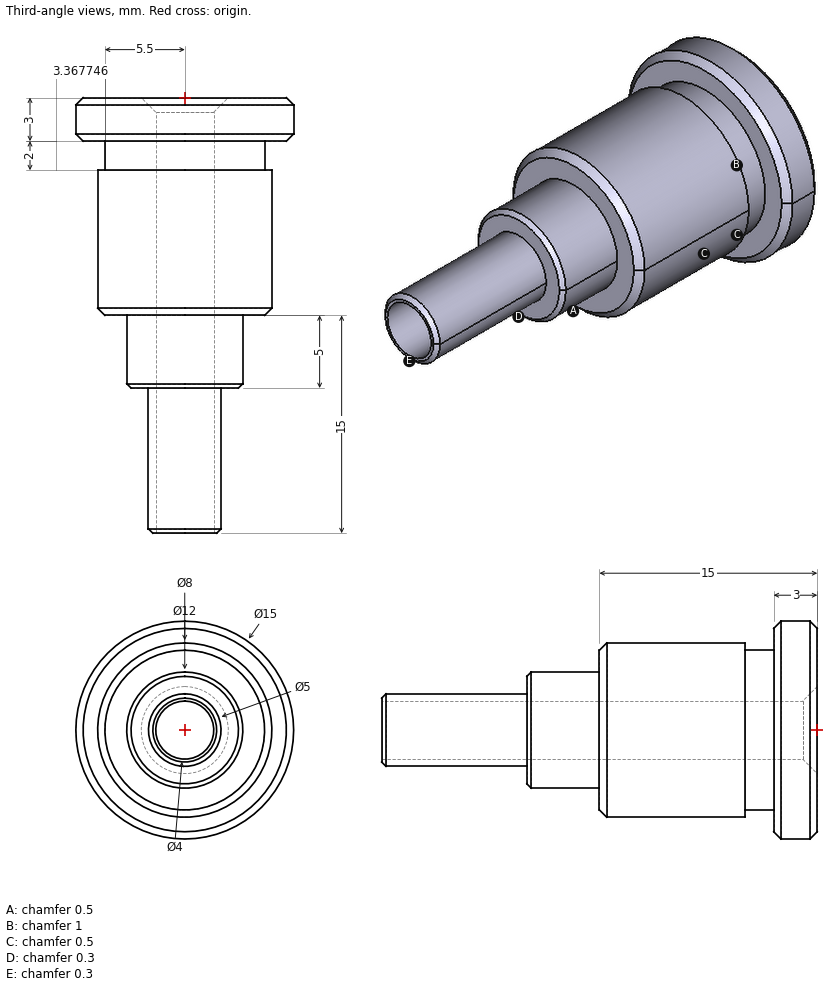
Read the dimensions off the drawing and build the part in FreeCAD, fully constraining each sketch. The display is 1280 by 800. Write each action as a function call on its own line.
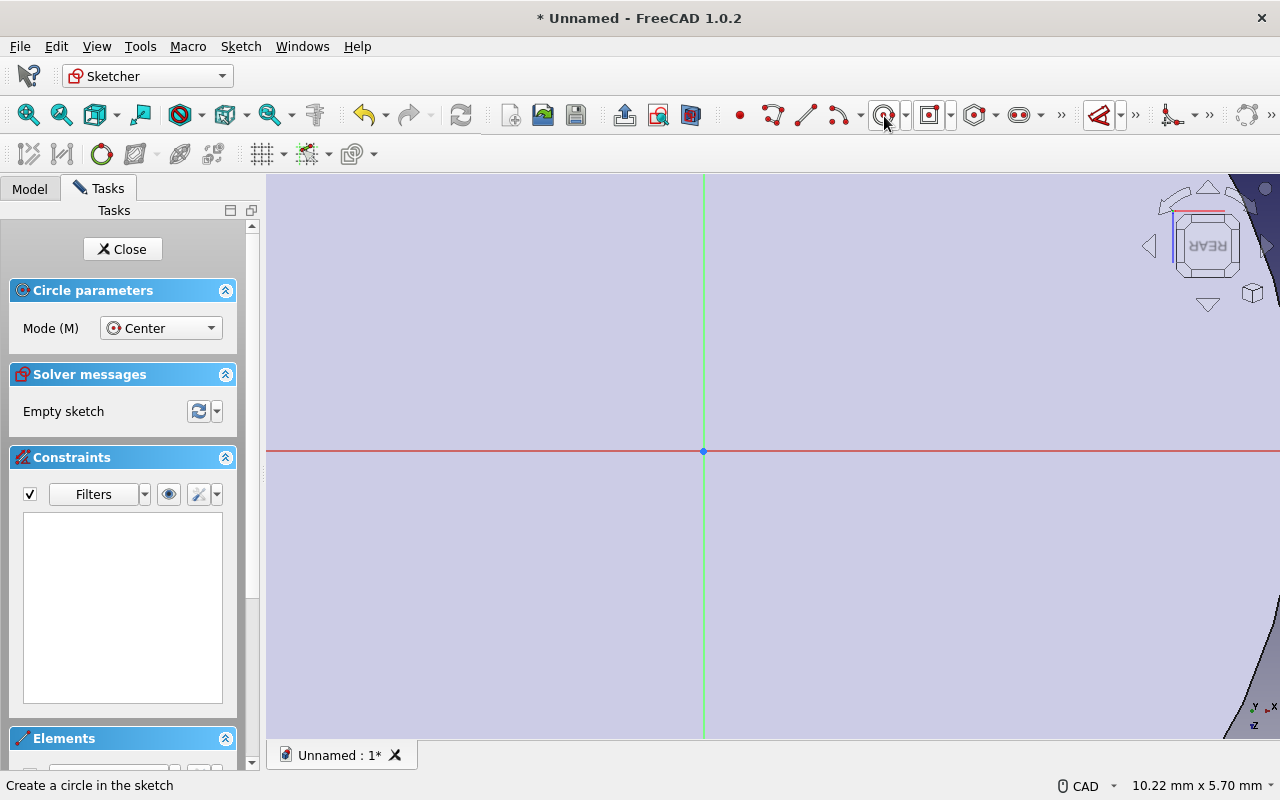
click(704, 451)
move(844, 311)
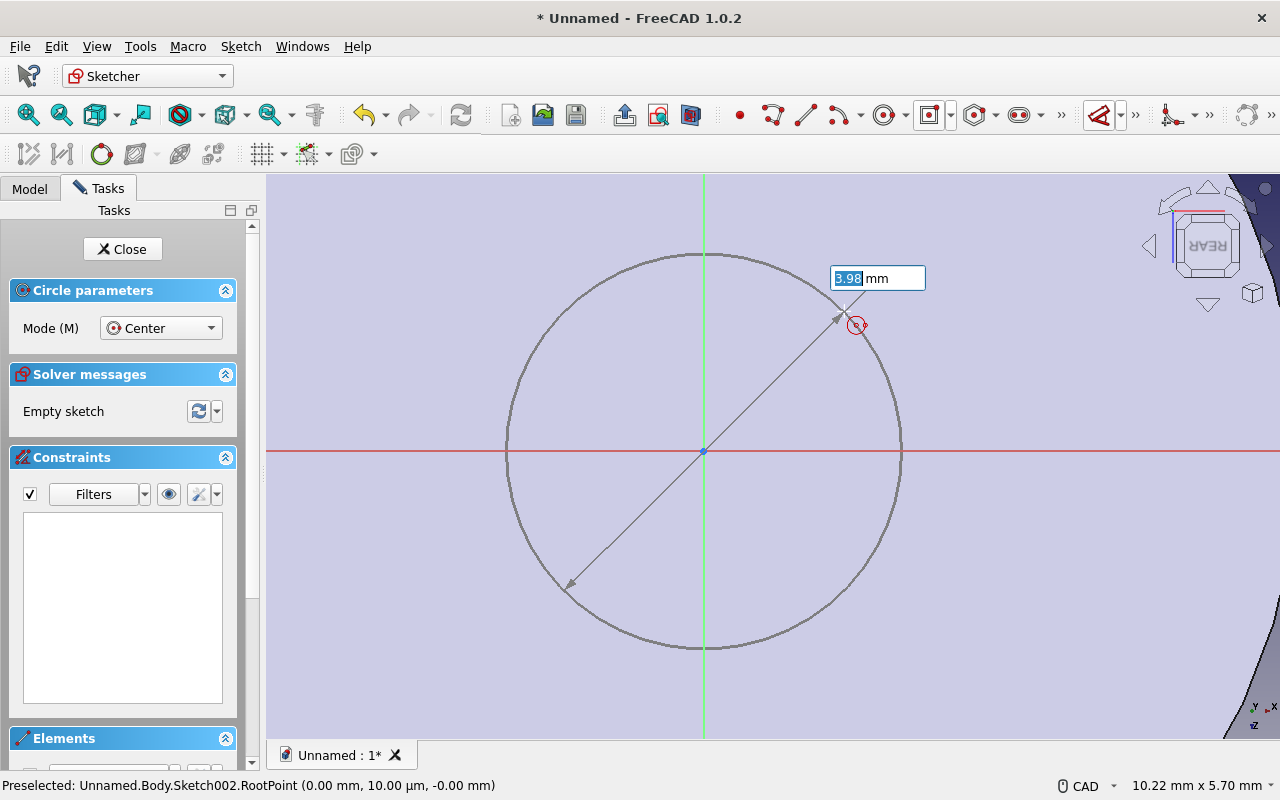
text(4)
key(Return)
key(Escape)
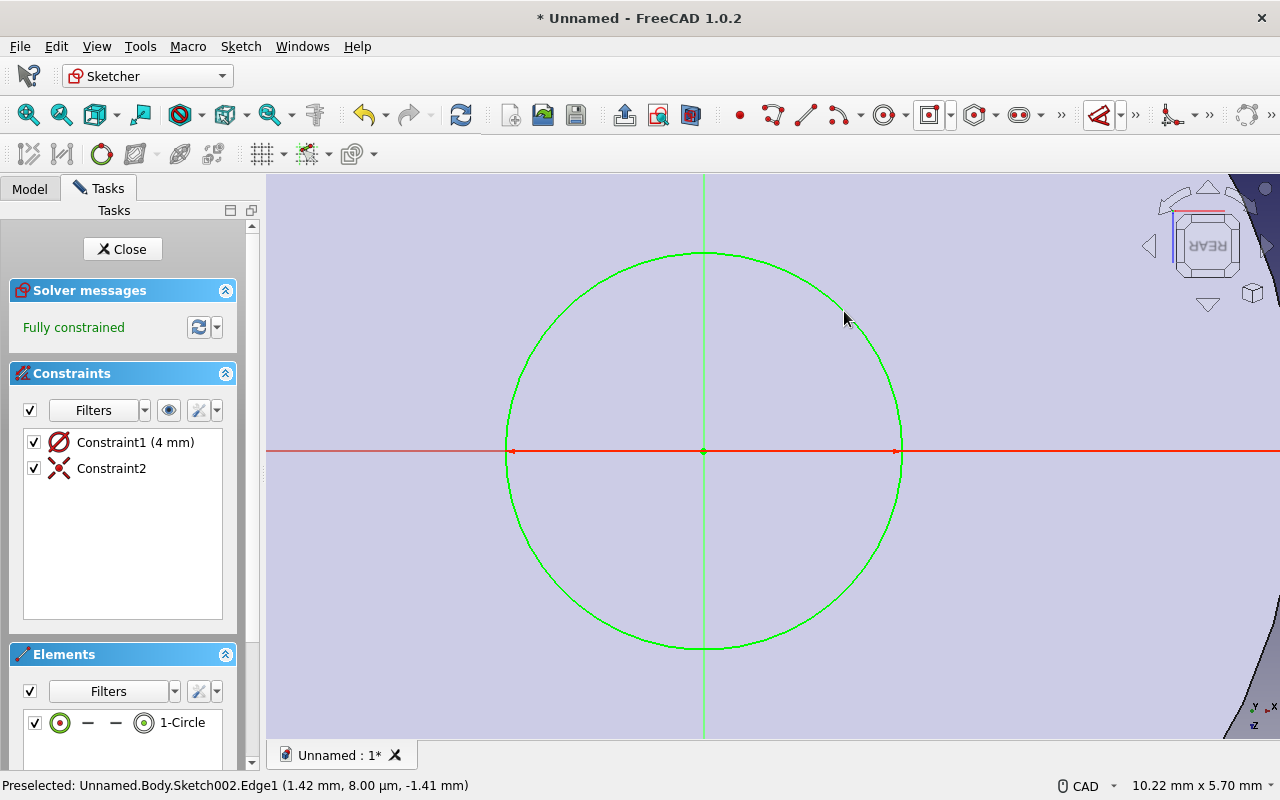
click(123, 249)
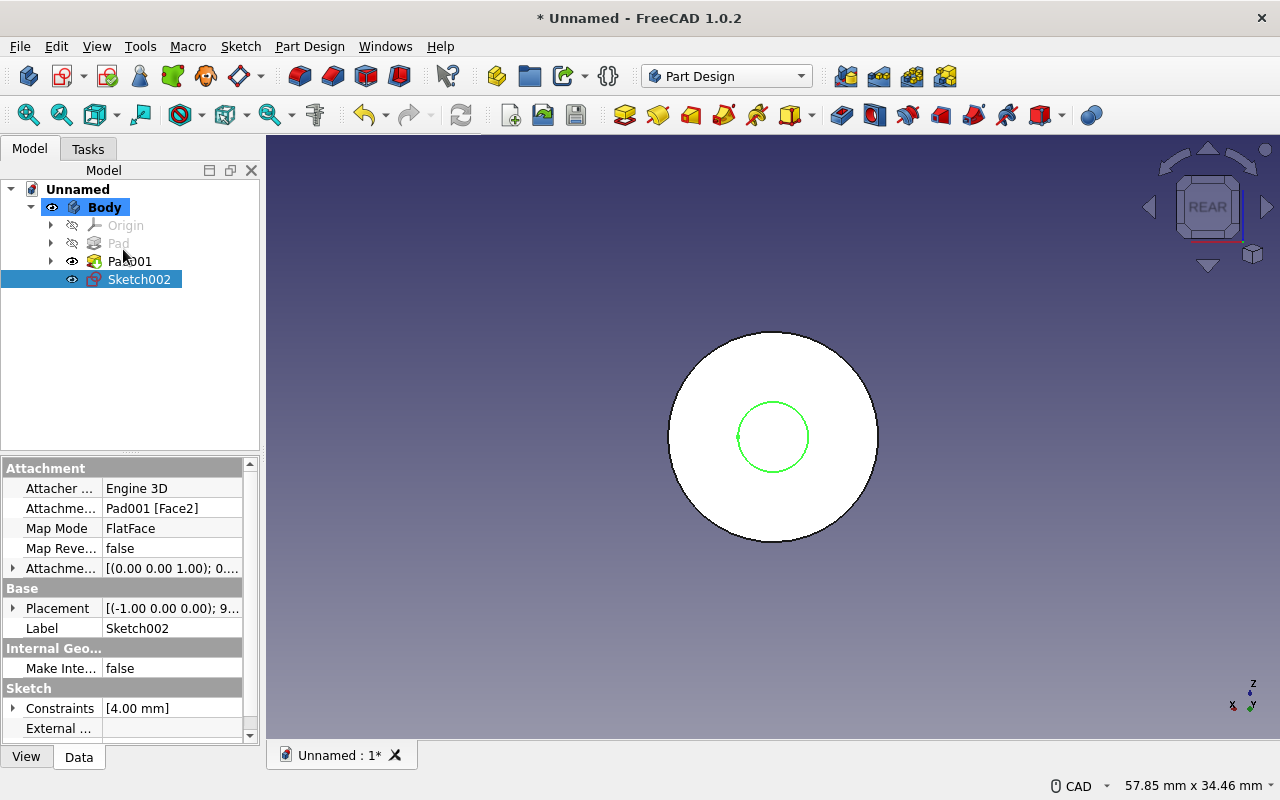
click(842, 116)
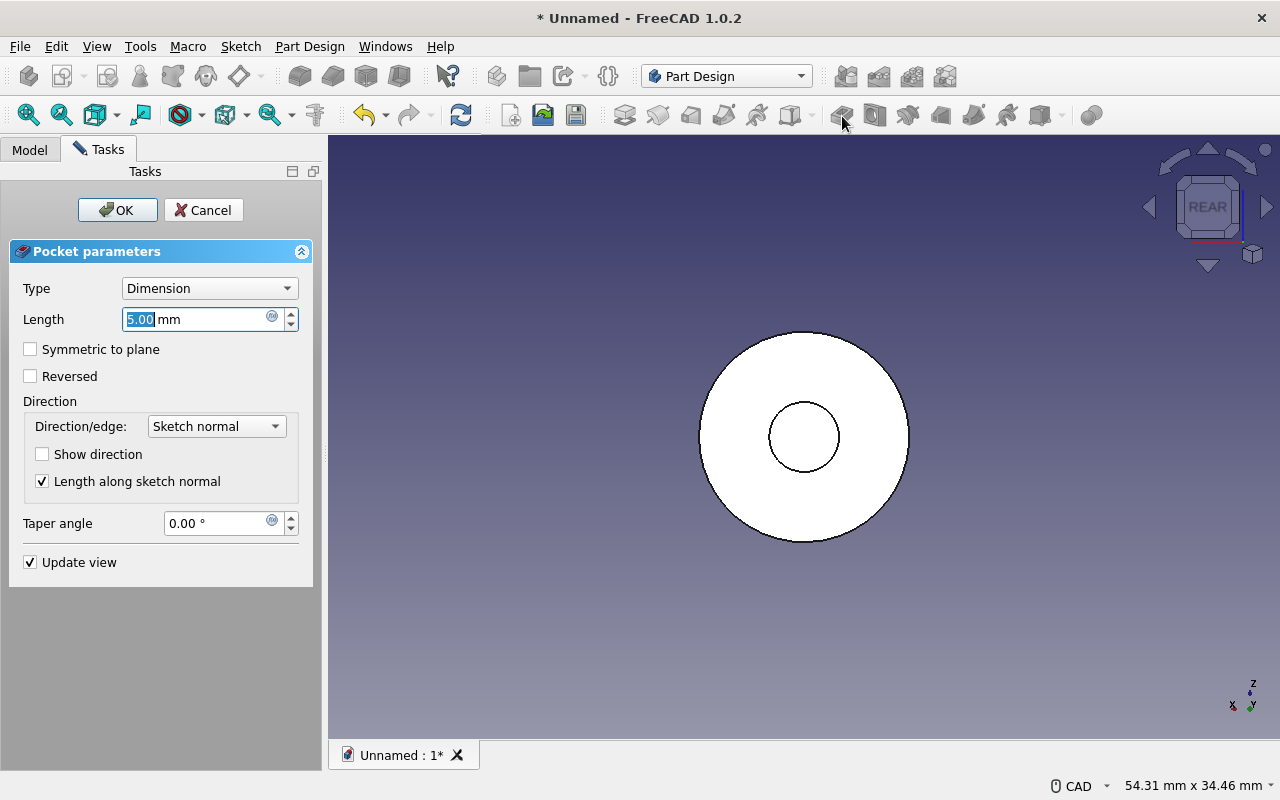
click(210, 288)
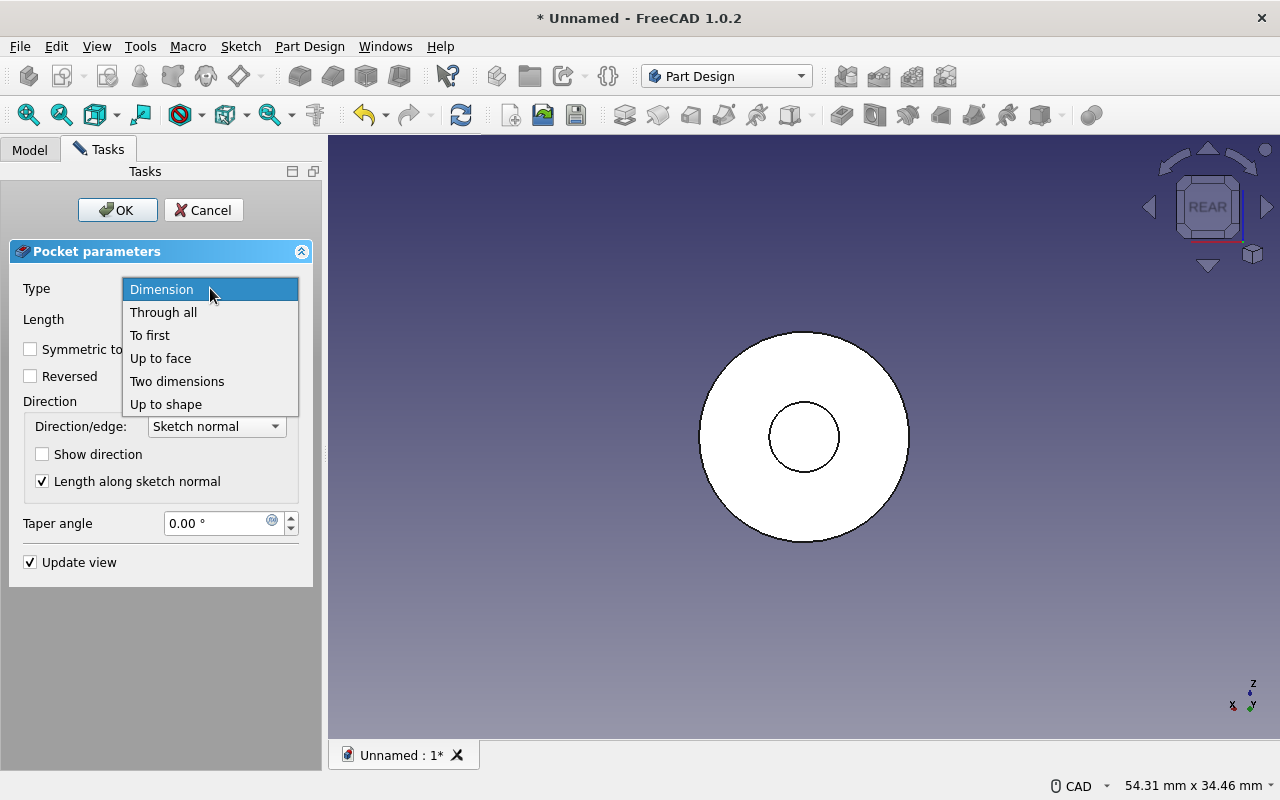
click(208, 312)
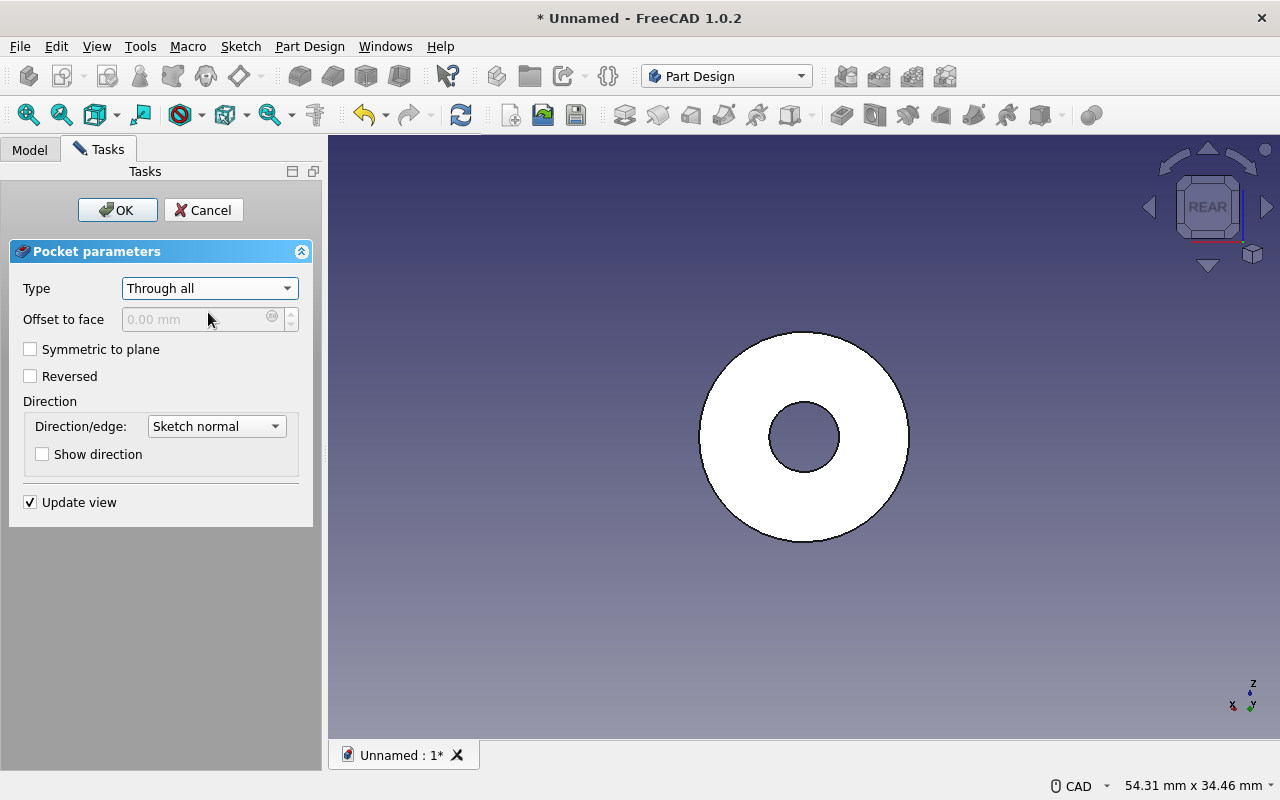
click(118, 210)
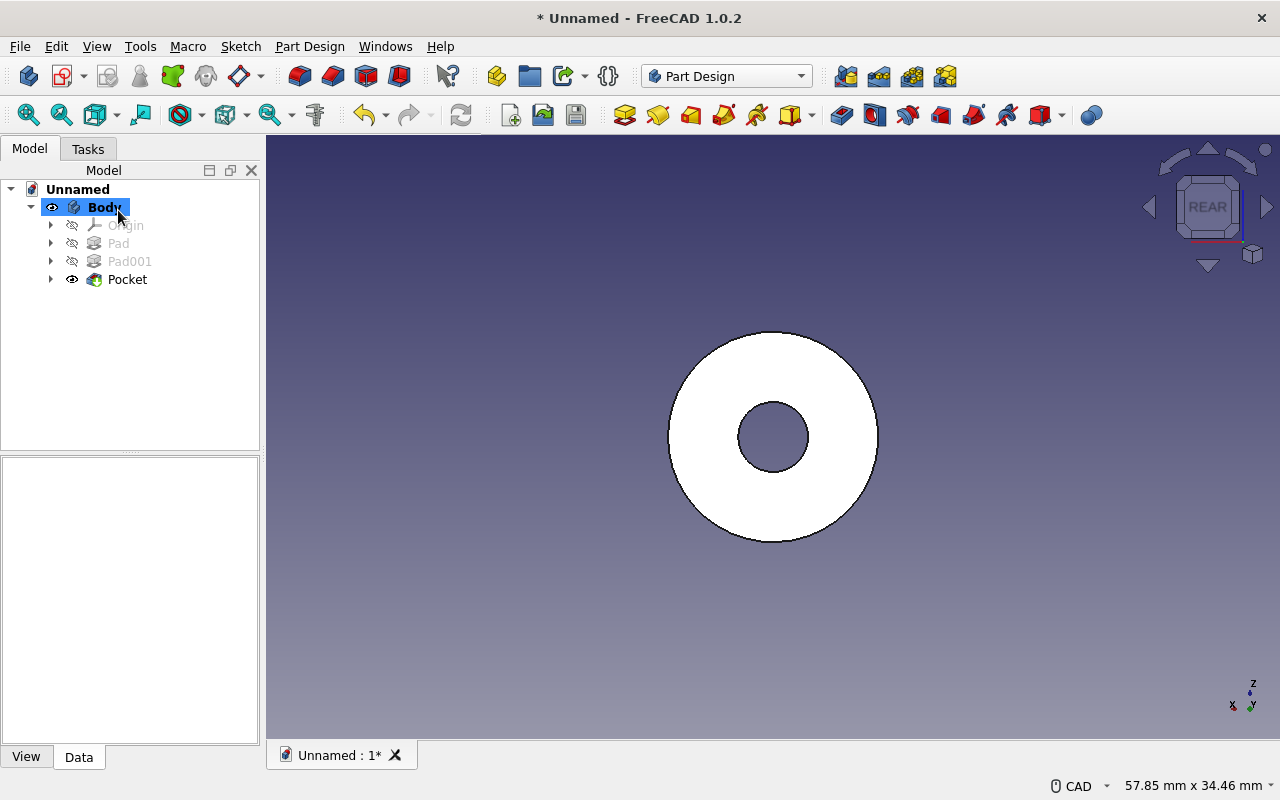
click(29, 116)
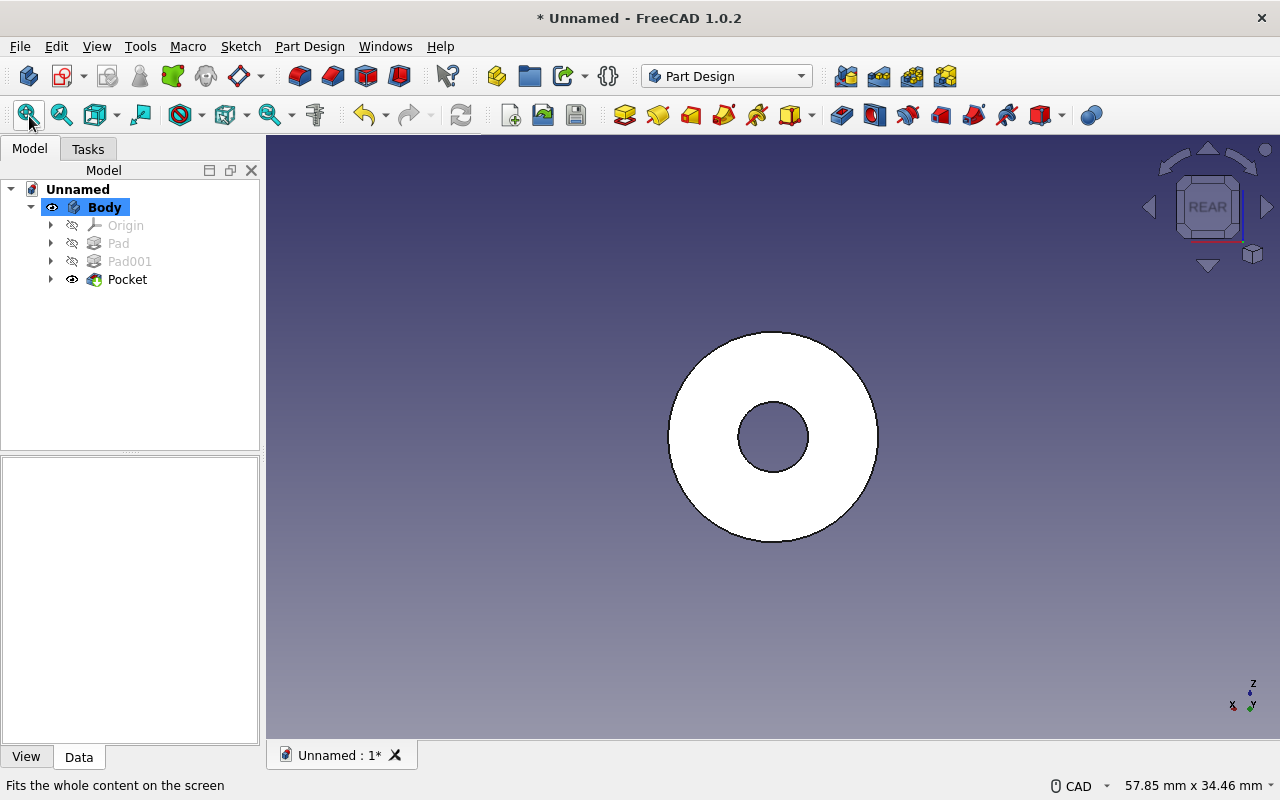
key(0)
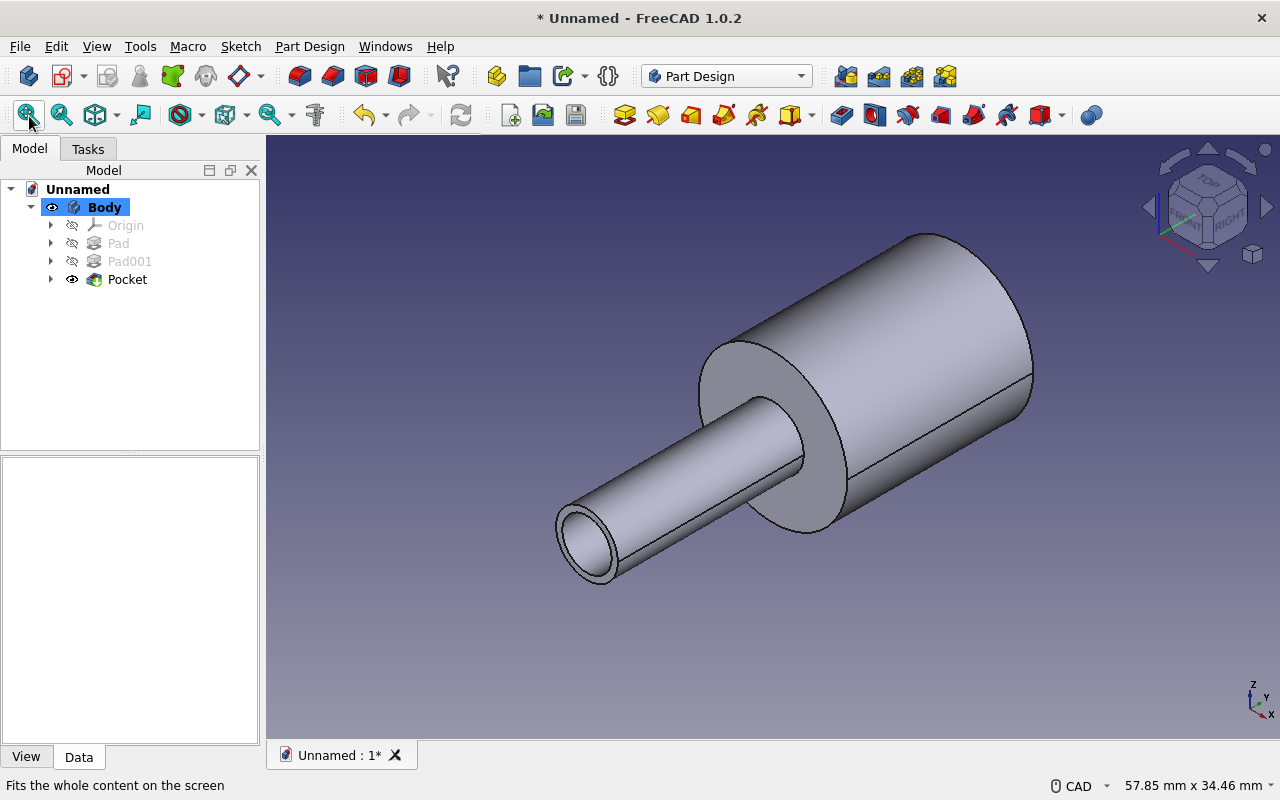
click(750, 341)